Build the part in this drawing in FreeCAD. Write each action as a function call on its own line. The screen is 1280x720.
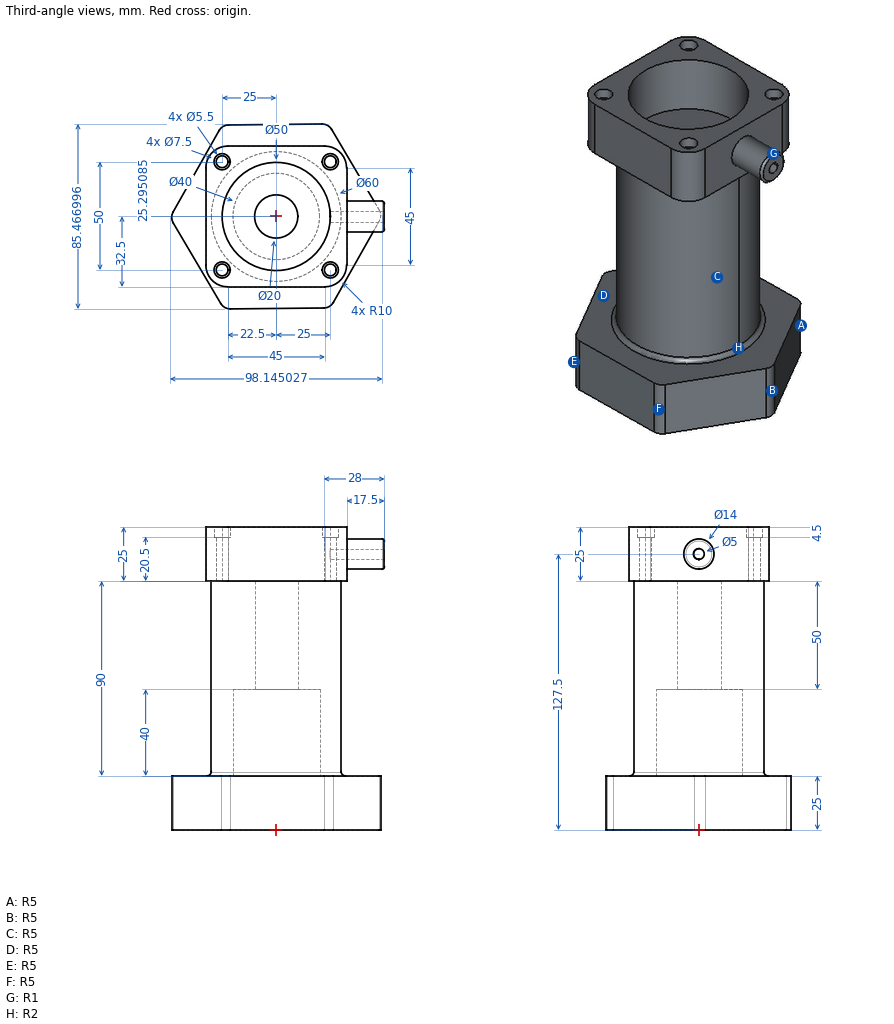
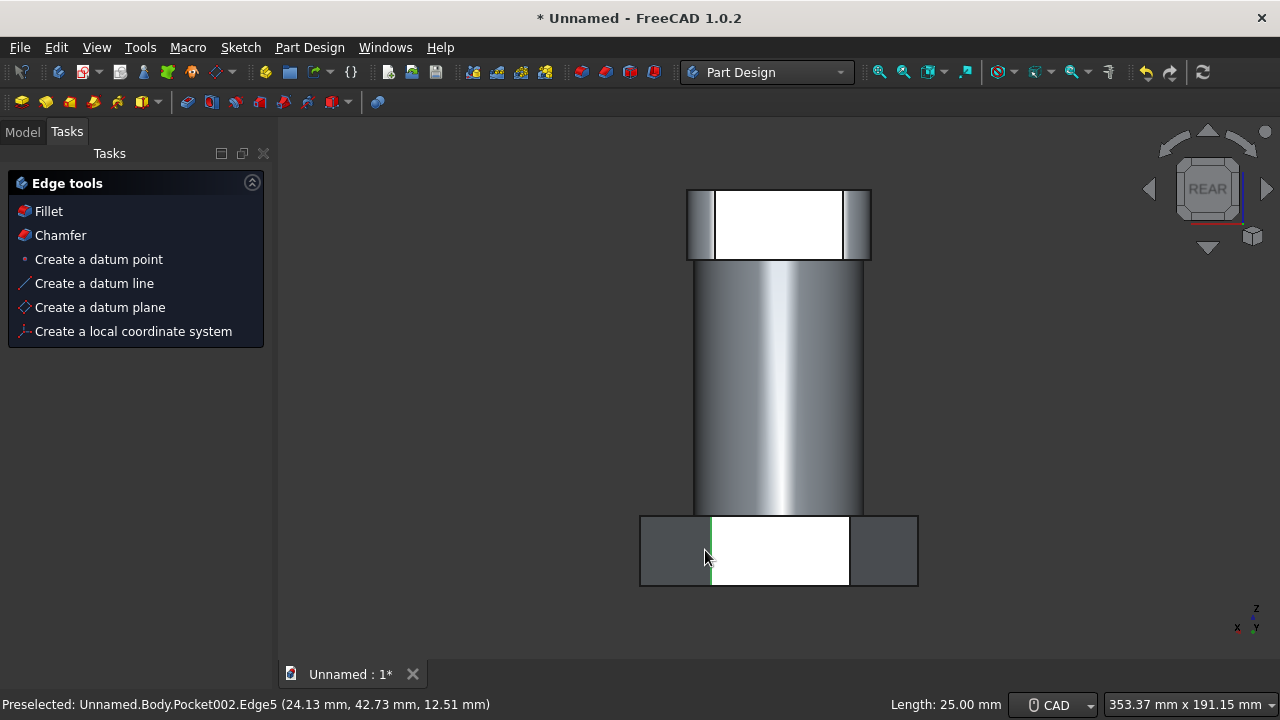
click(582, 72)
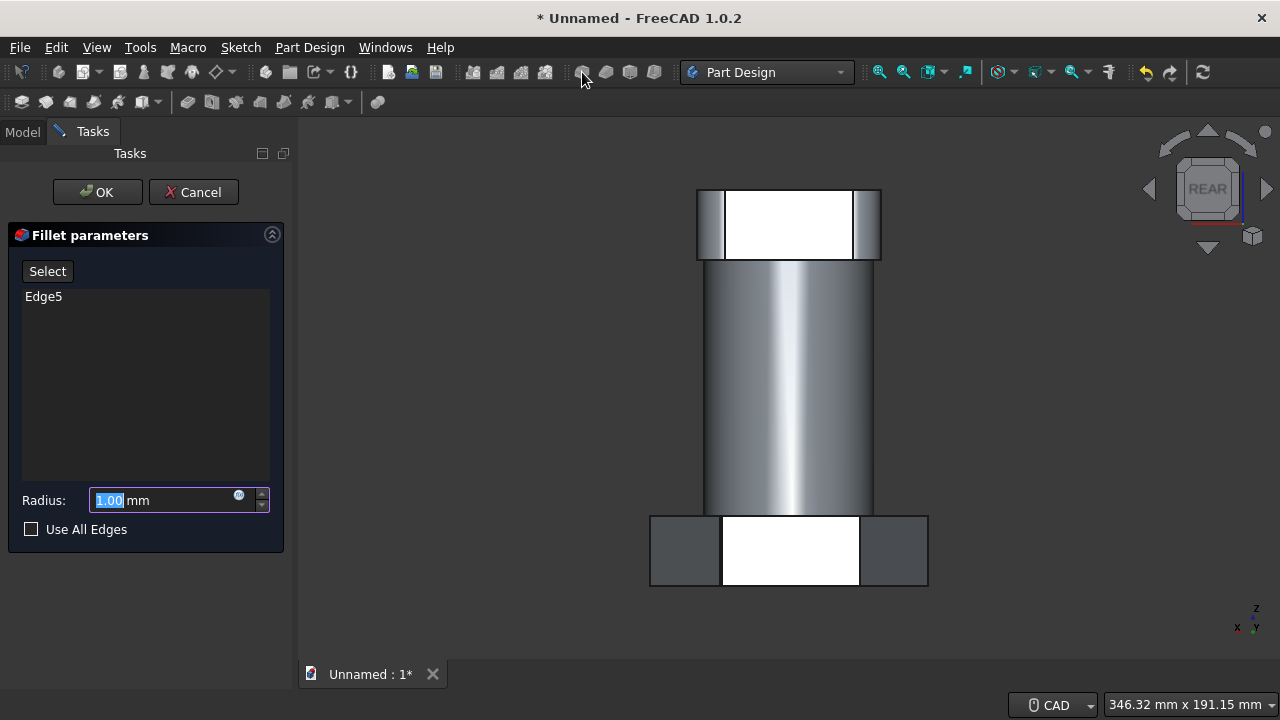
text(5)
key(Tab)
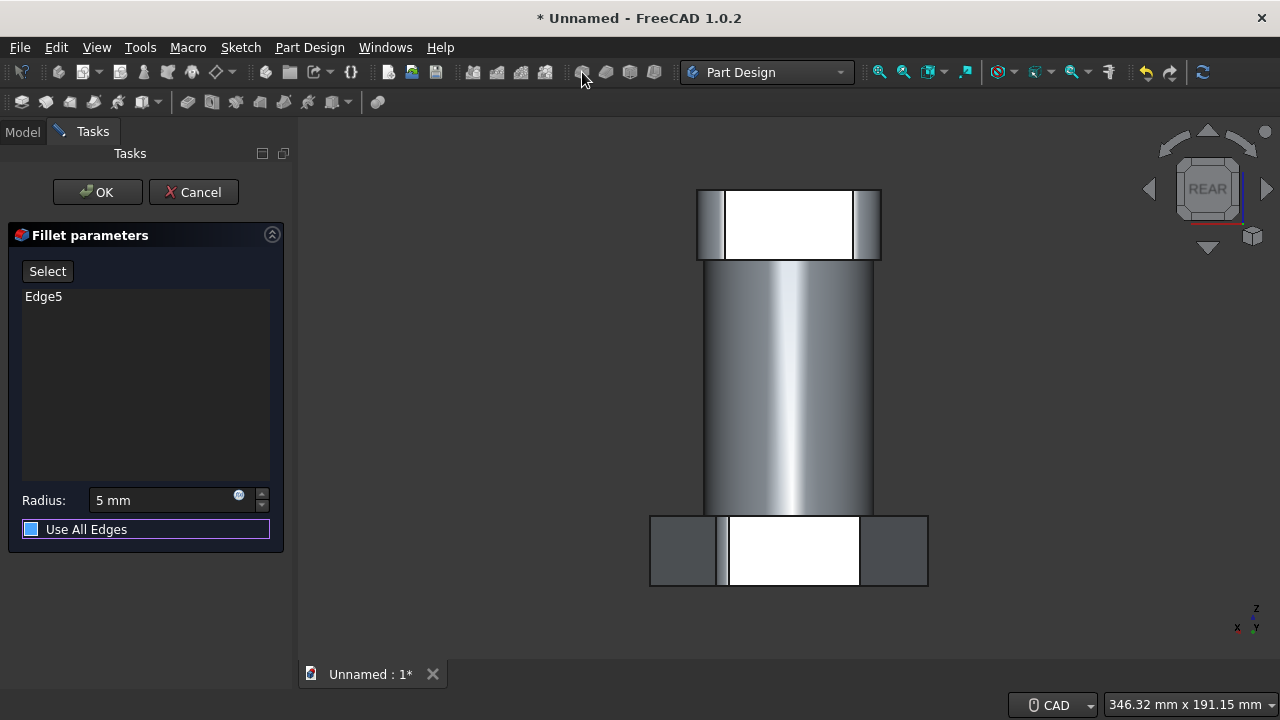
click(98, 192)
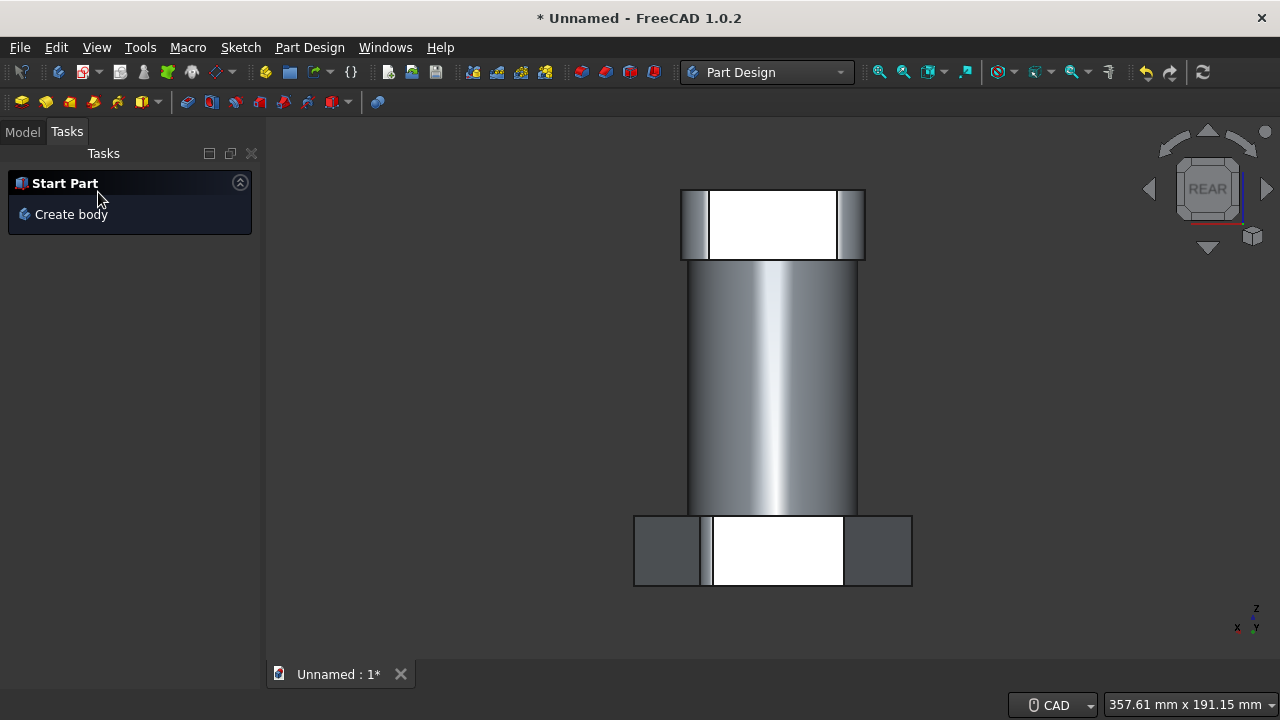
key(0)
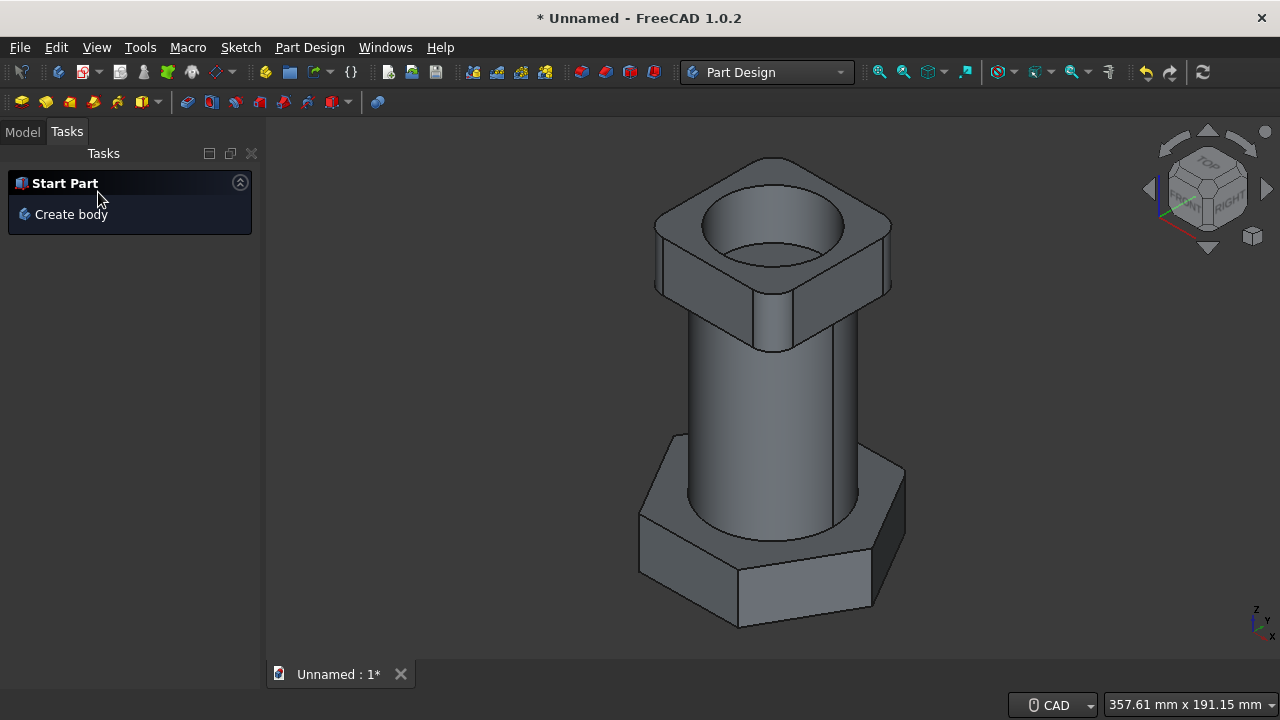
key(2)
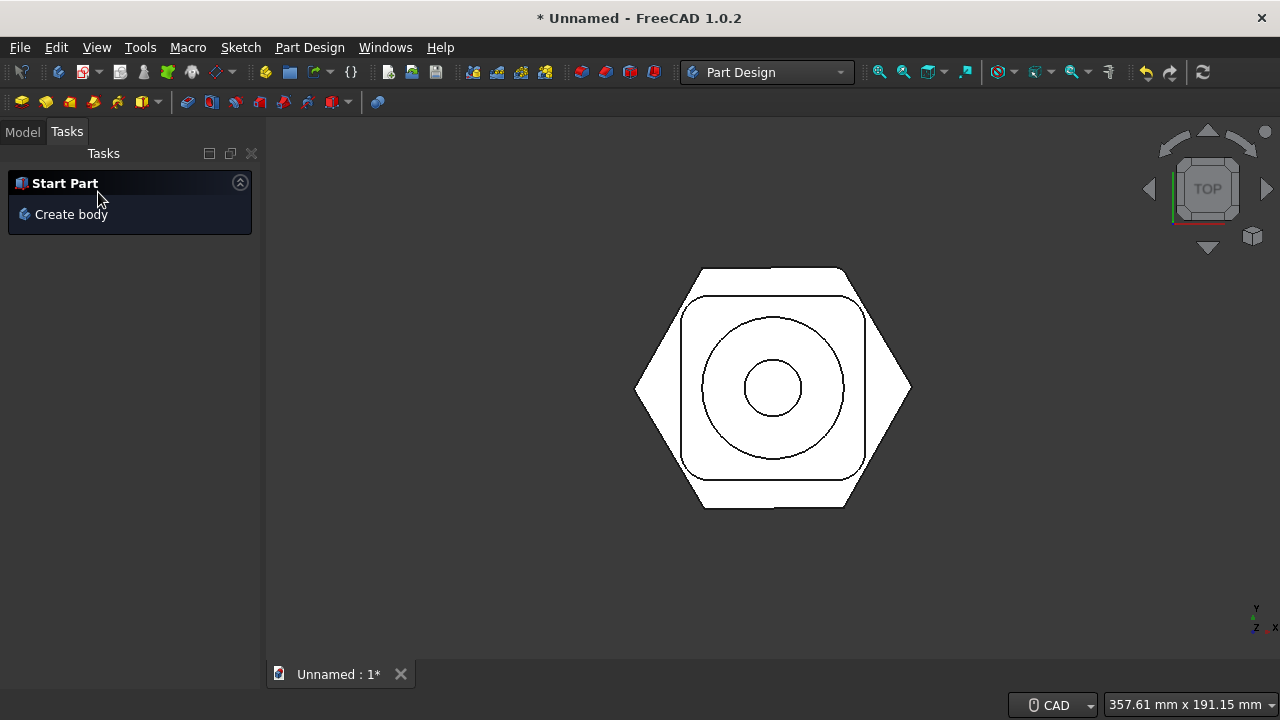
click(880, 72)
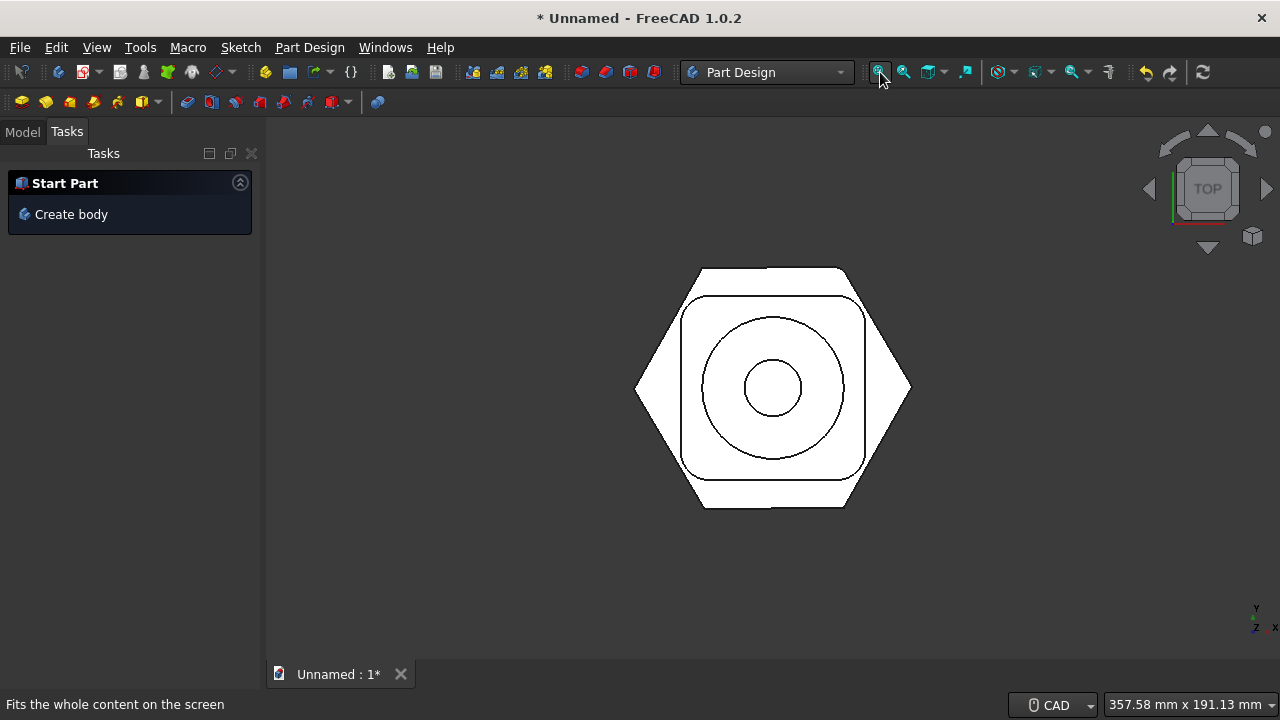
key(1)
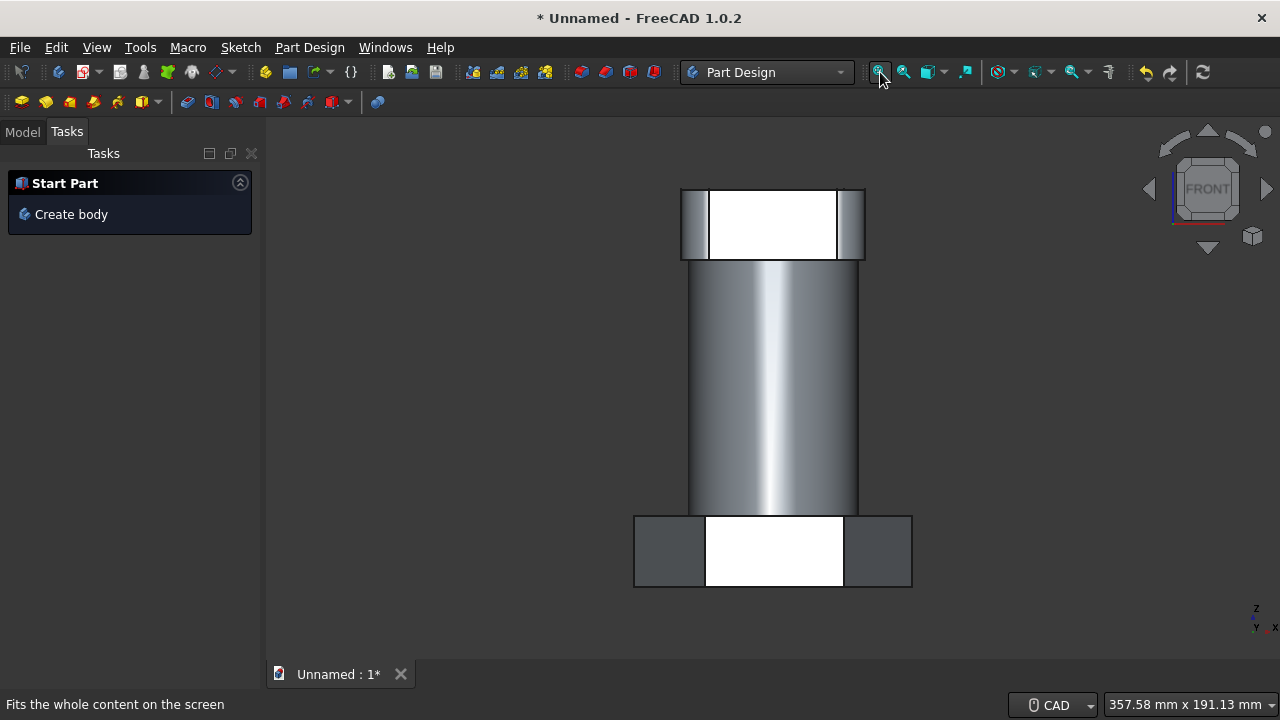
key(3)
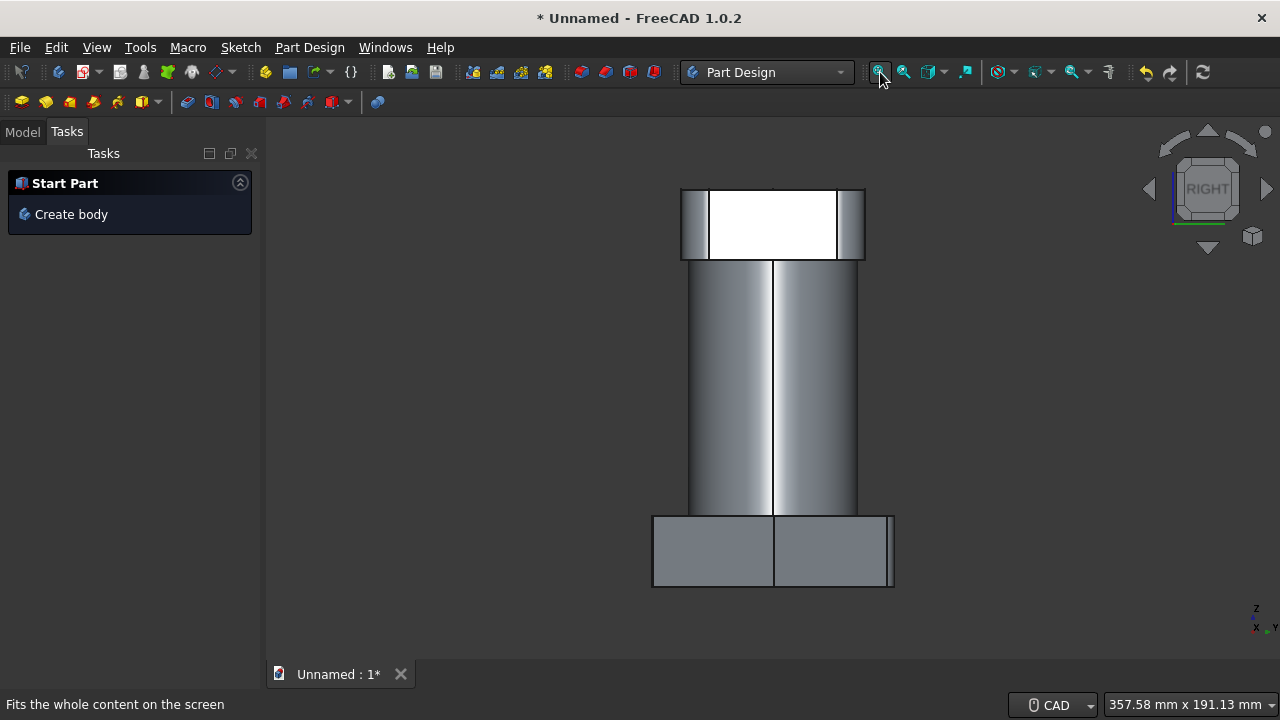
click(774, 550)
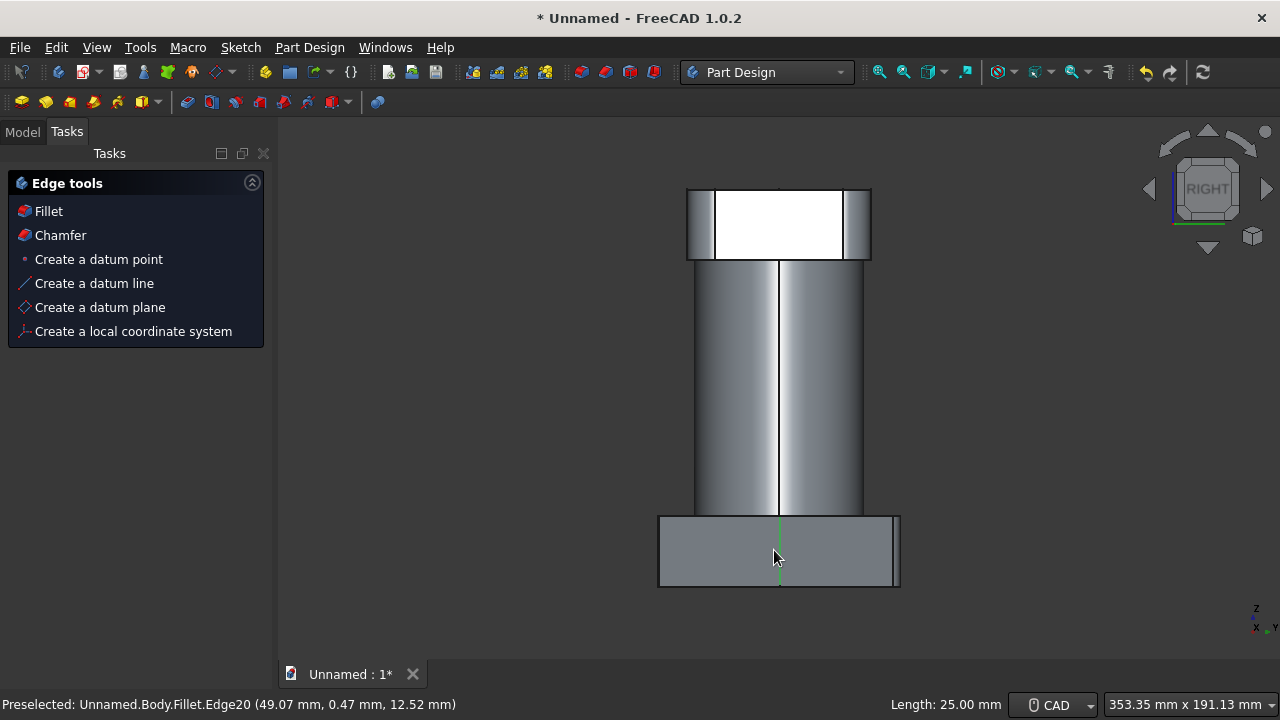
click(582, 72)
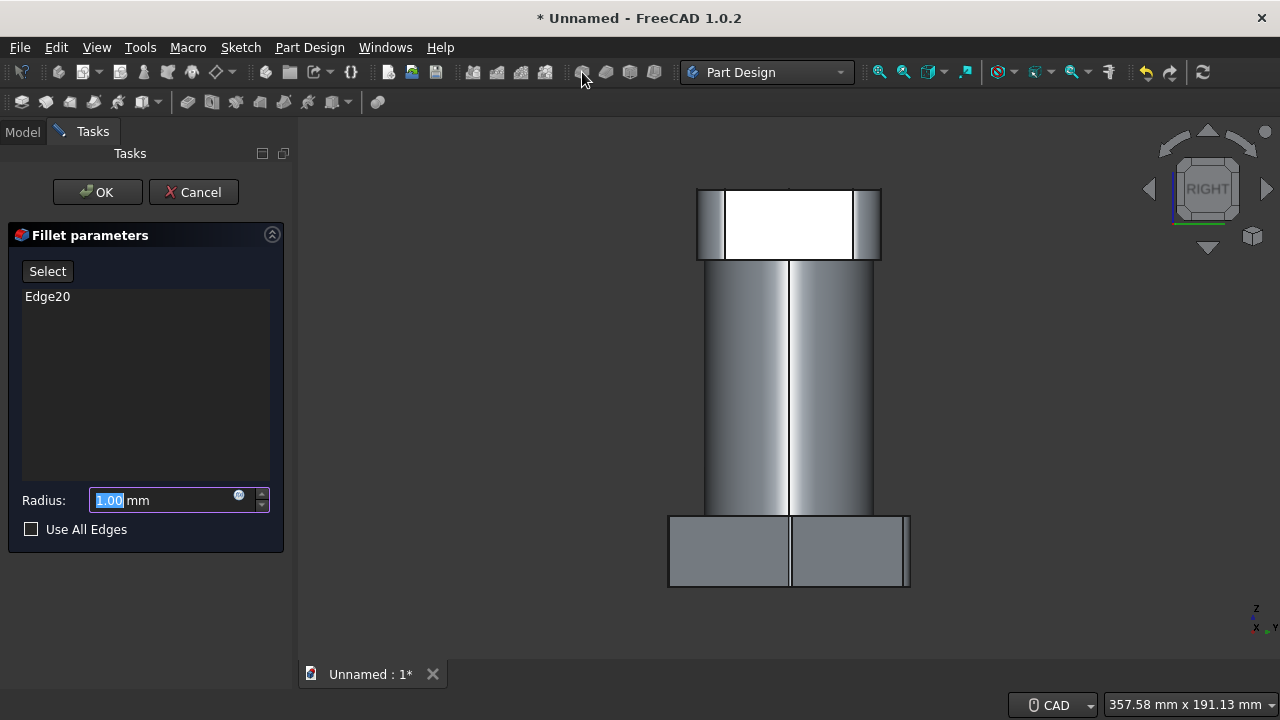
text(5)
key(Tab)